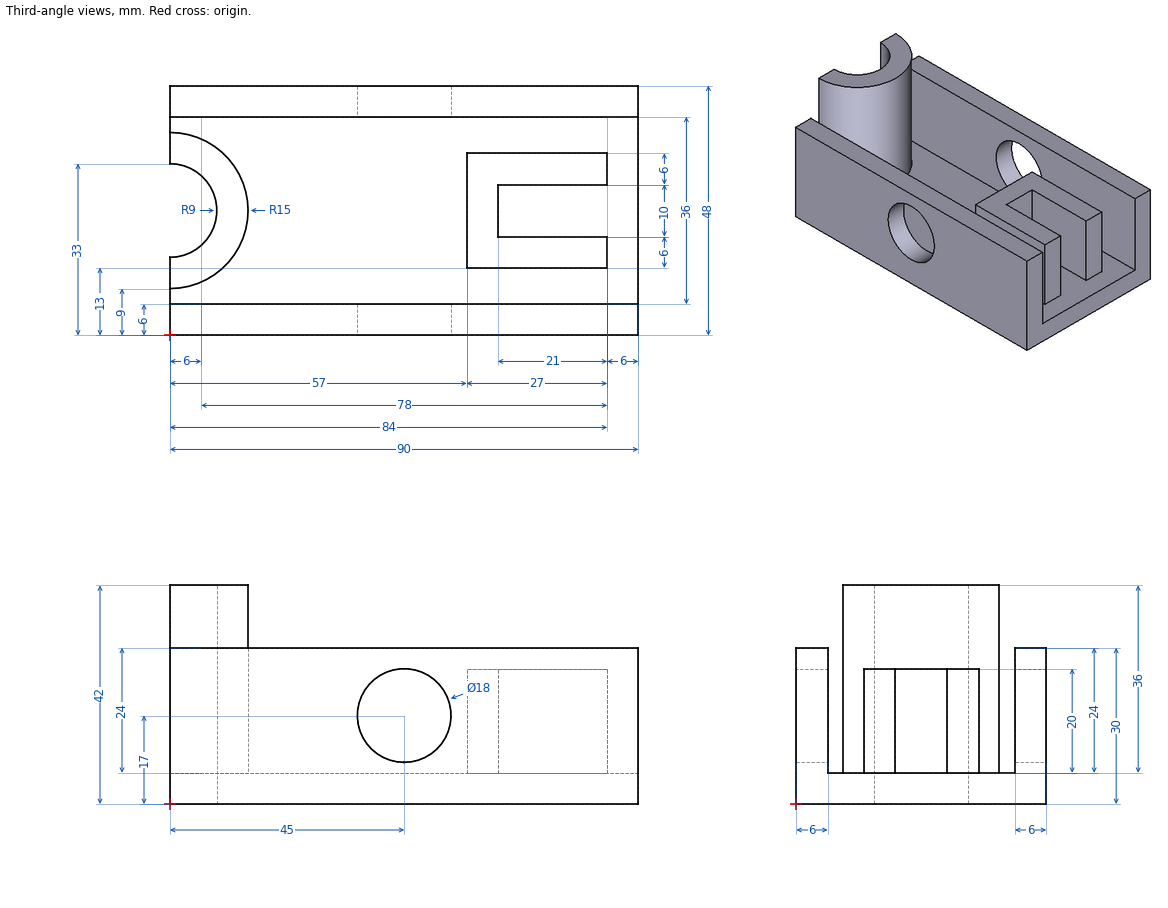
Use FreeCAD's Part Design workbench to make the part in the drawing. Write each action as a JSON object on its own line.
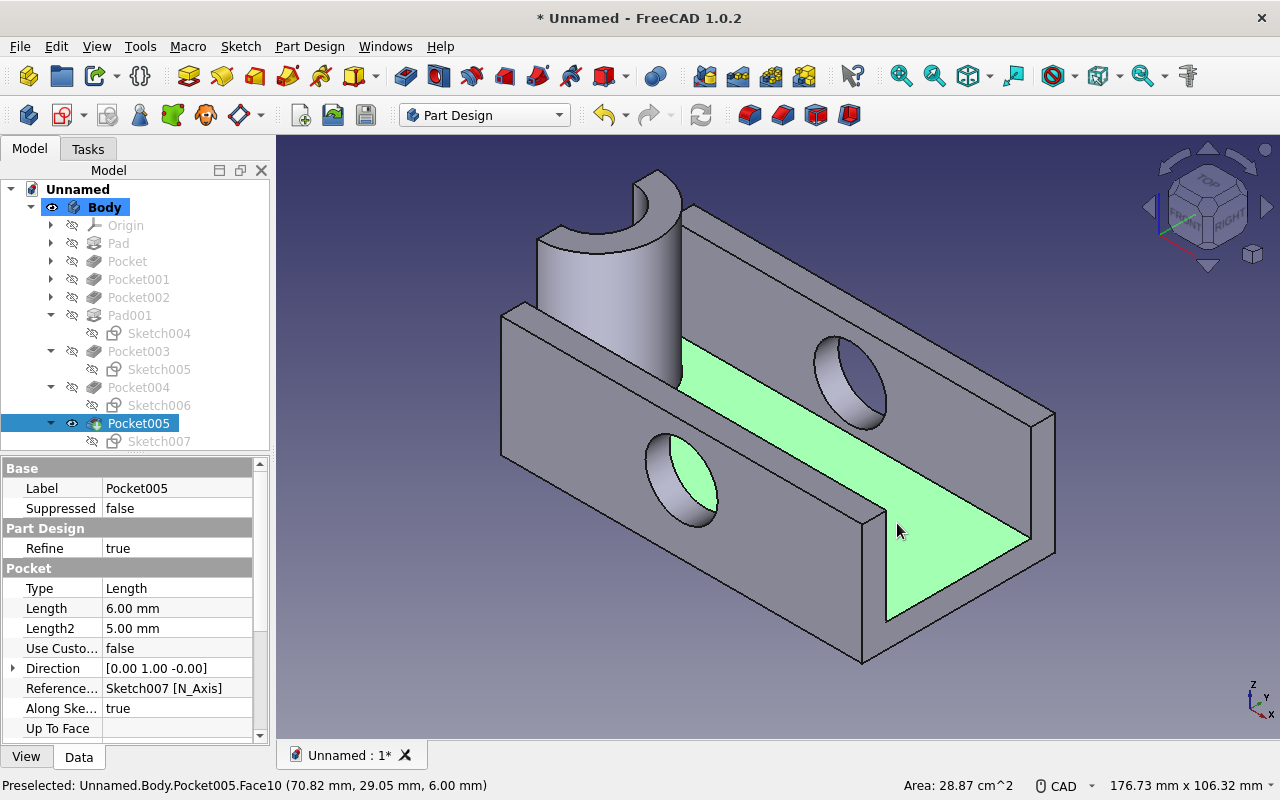
{"action": "left_click", "coordinate": [62, 116]}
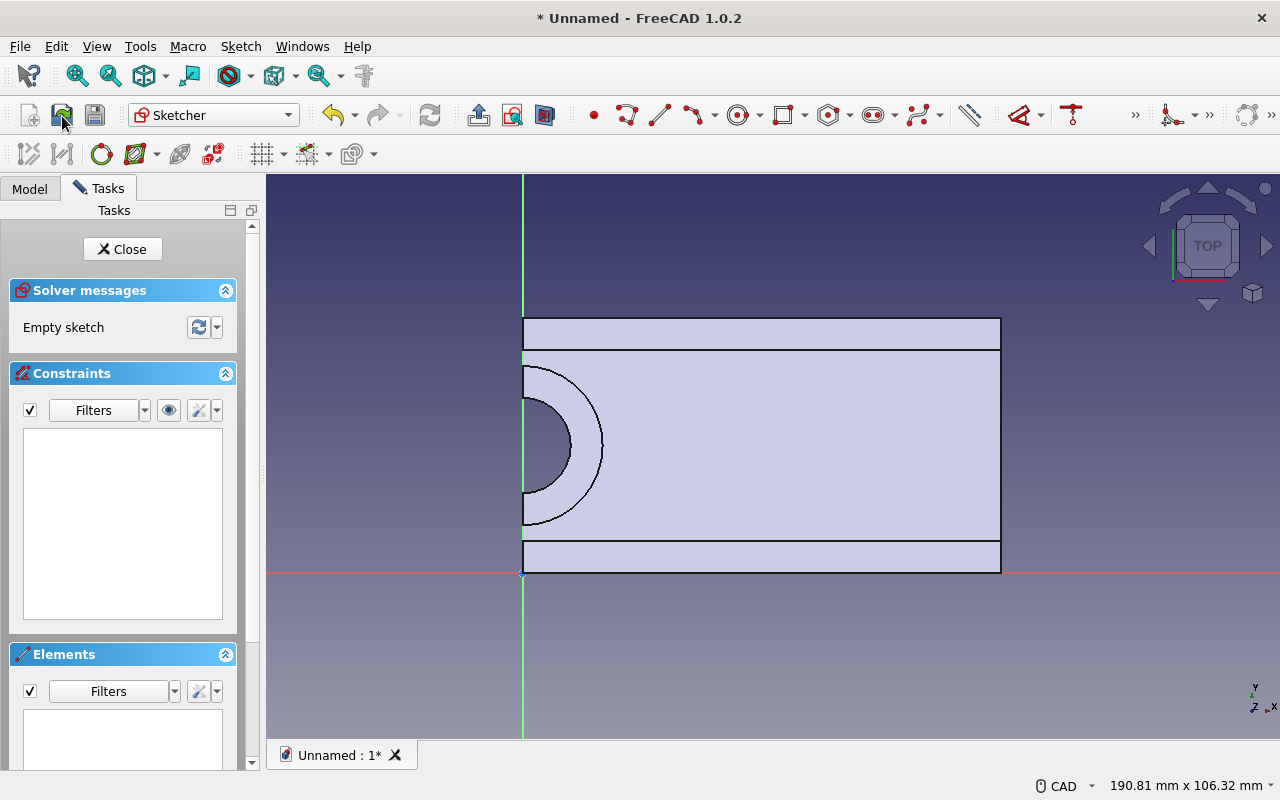
{"action": "scroll", "coordinate": [981, 441], "scroll_direction": "up", "scroll_amount": 6}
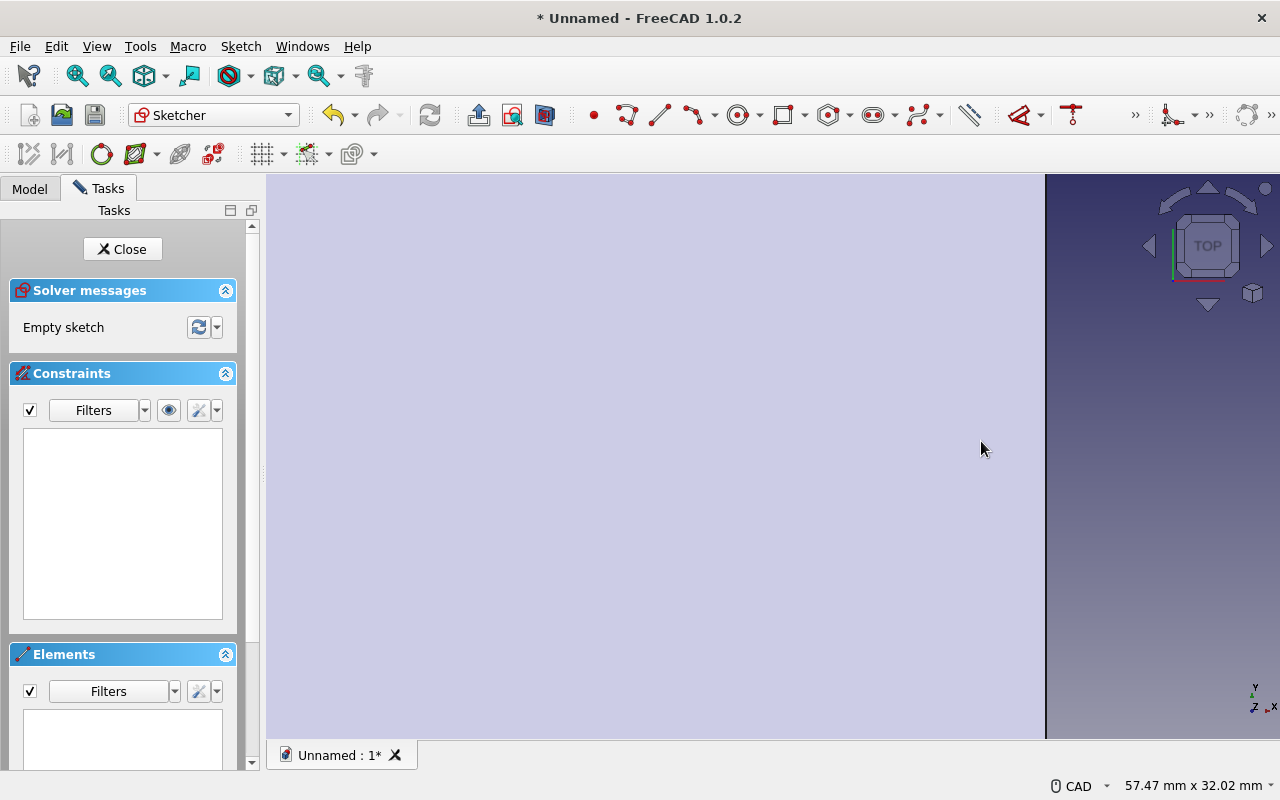
{"action": "key", "text": "g m"}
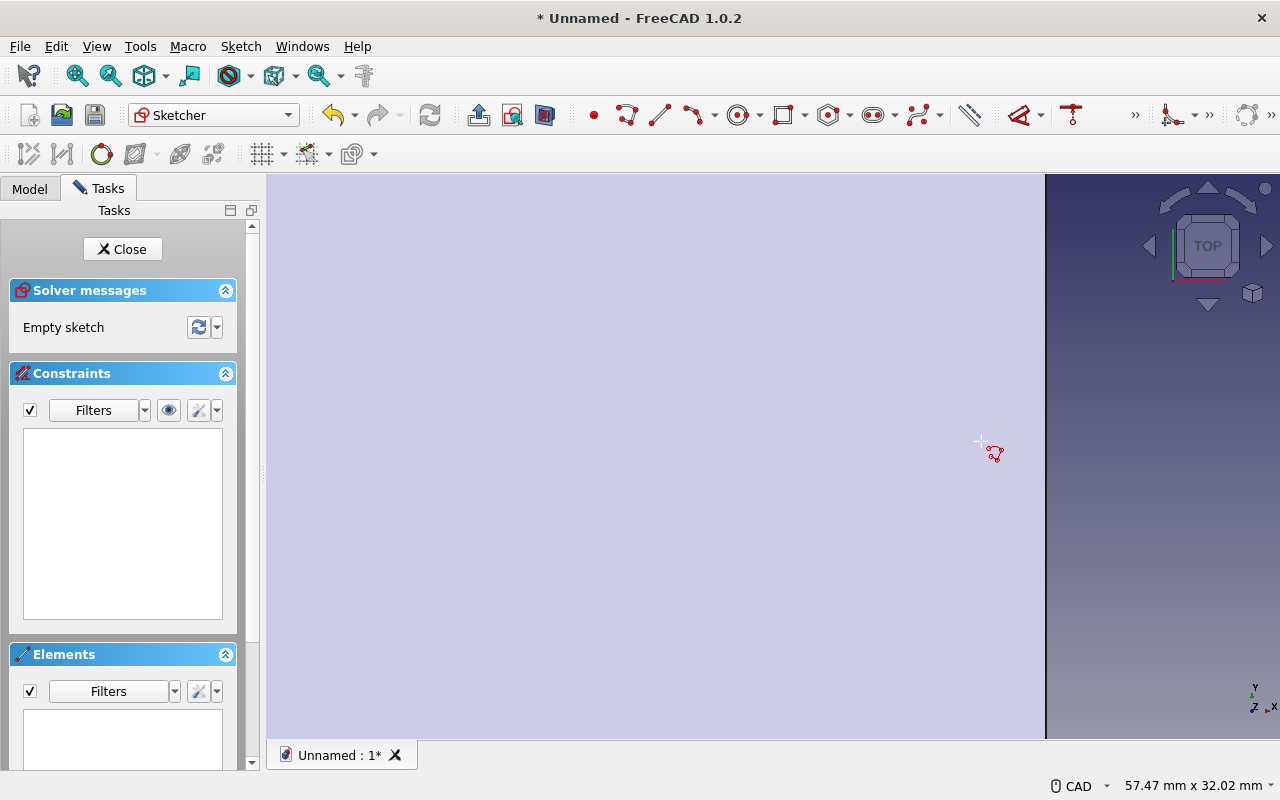
{"action": "left_click", "coordinate": [464, 649]}
{"action": "left_click", "coordinate": [941, 649]}
{"action": "left_click", "coordinate": [941, 543]}
{"action": "left_click", "coordinate": [570, 543]}
{"action": "left_click", "coordinate": [570, 367]}
{"action": "left_click", "coordinate": [941, 367]}
{"action": "left_click", "coordinate": [941, 261]}
{"action": "left_click", "coordinate": [464, 261]}
{"action": "left_click", "coordinate": [464, 650]}
{"action": "key", "text": "Escape"}
{"action": "key", "text": "Escape"}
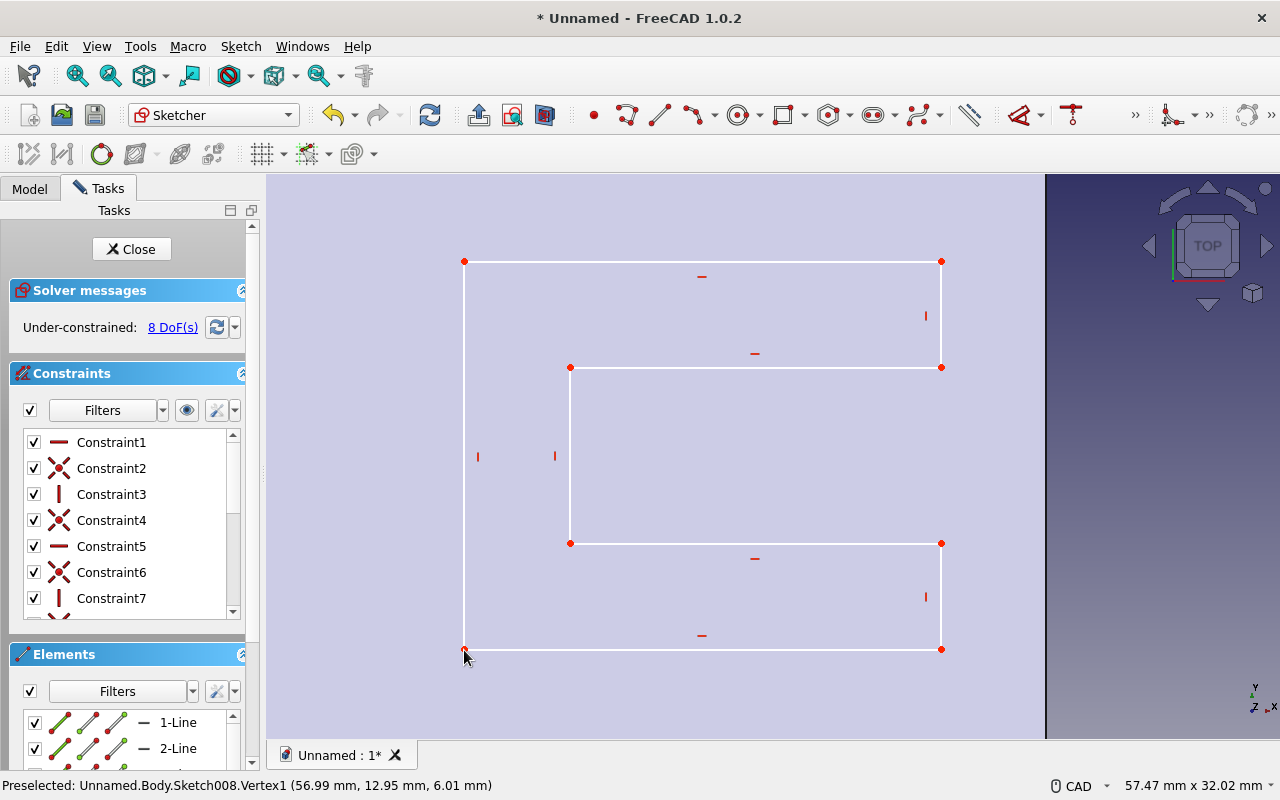
{"action": "left_click", "coordinate": [1018, 116]}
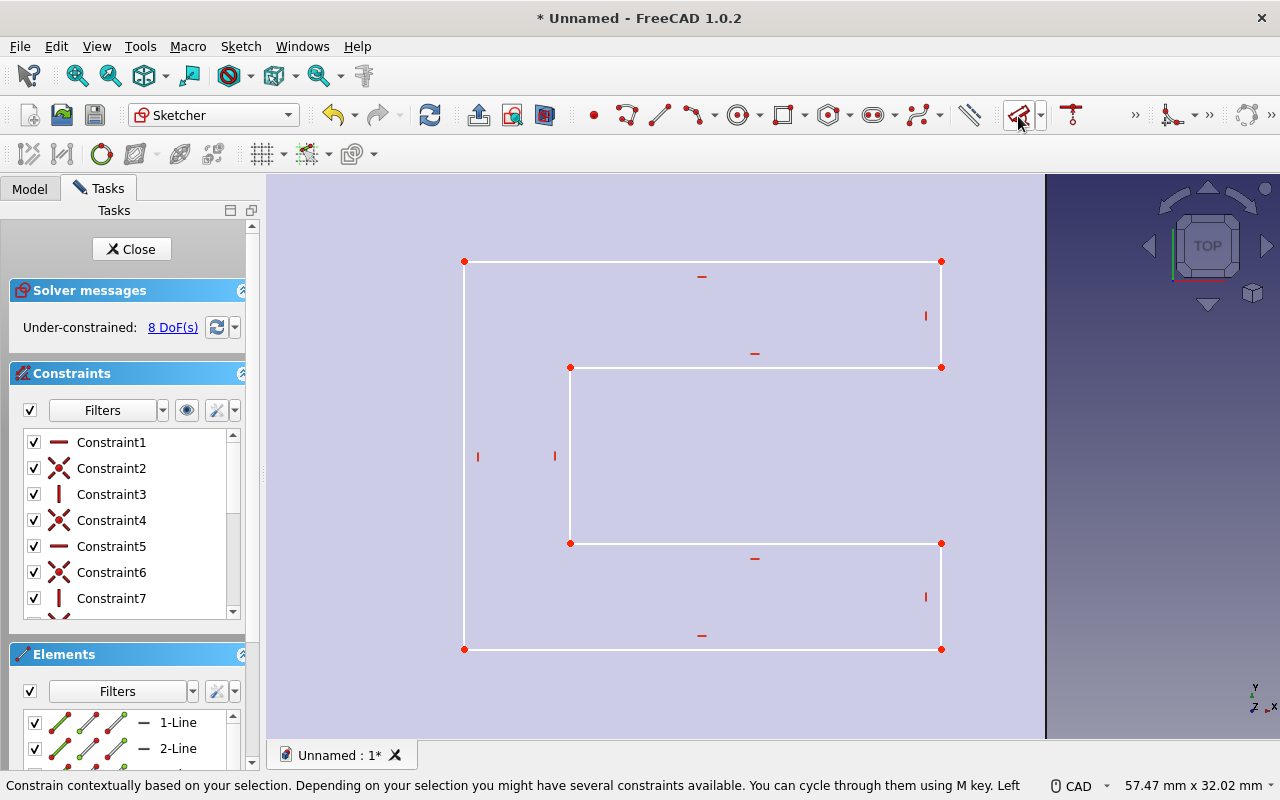
{"action": "left_click", "coordinate": [941, 618]}
{"action": "left_click", "coordinate": [975, 597]}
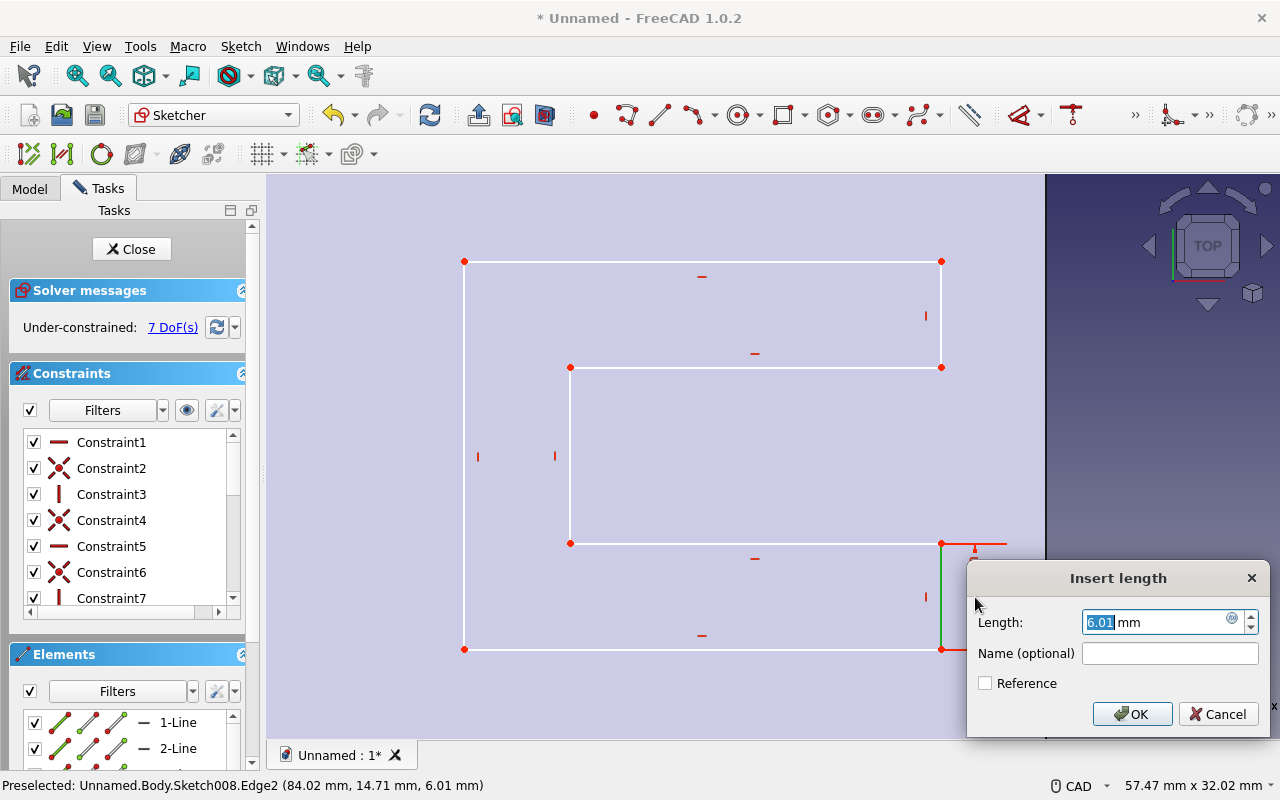
{"action": "type", "text": "6"}
{"action": "key", "text": "Return"}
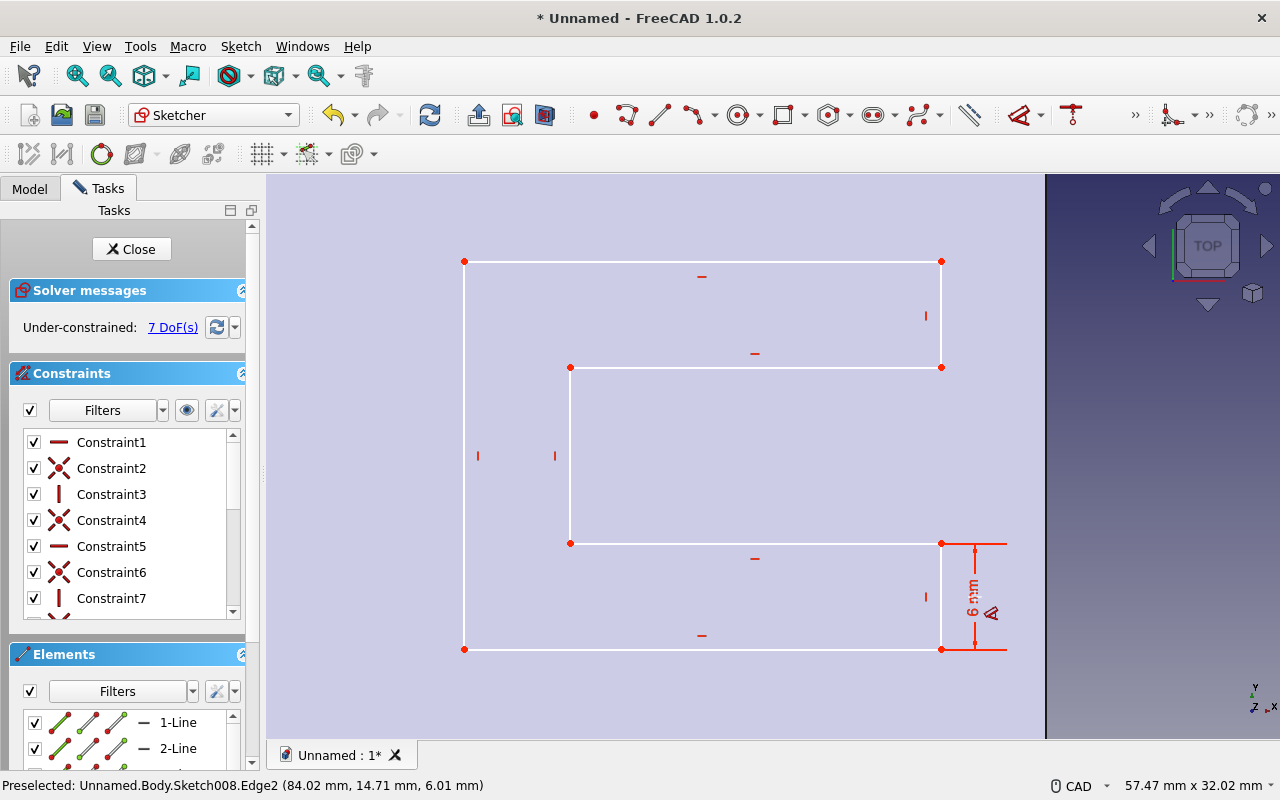
{"action": "left_click", "coordinate": [941, 336]}
{"action": "left_click", "coordinate": [975, 315]}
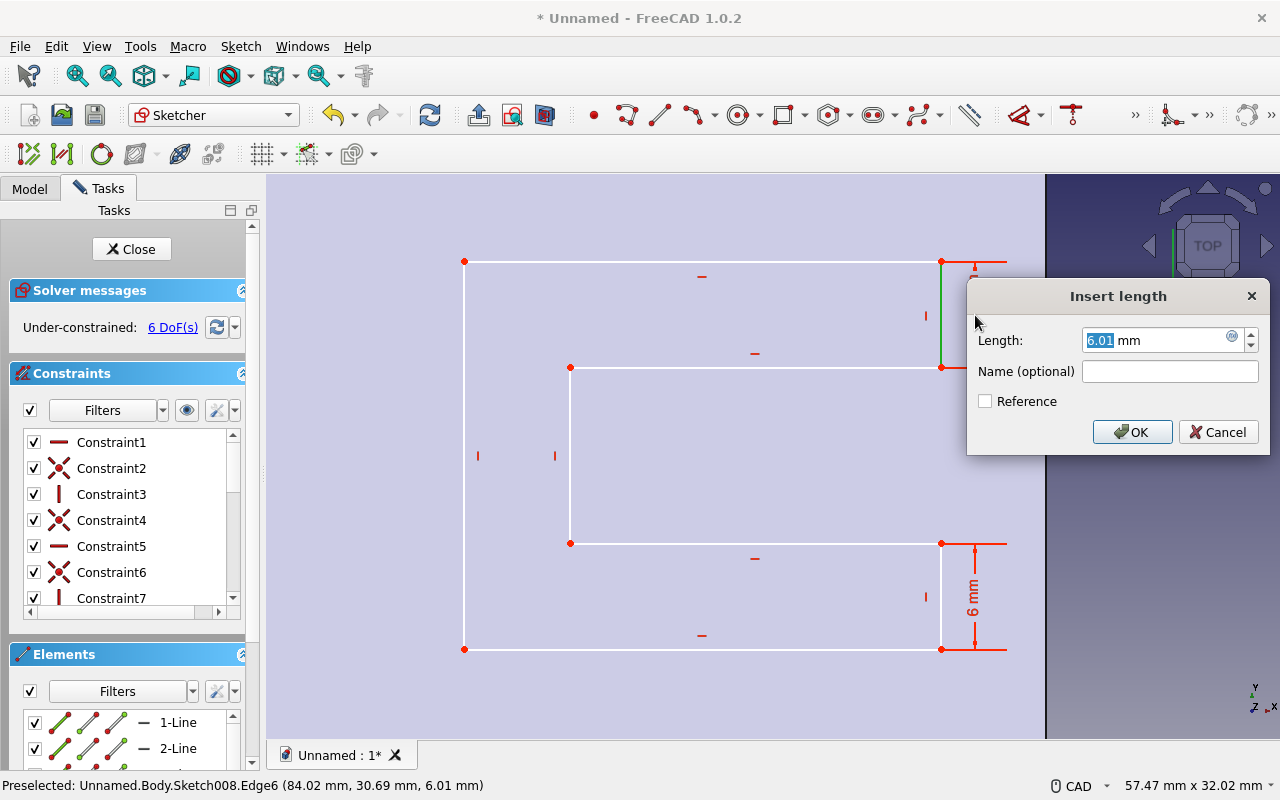
{"action": "type", "text": "6"}
{"action": "key", "text": "Return"}